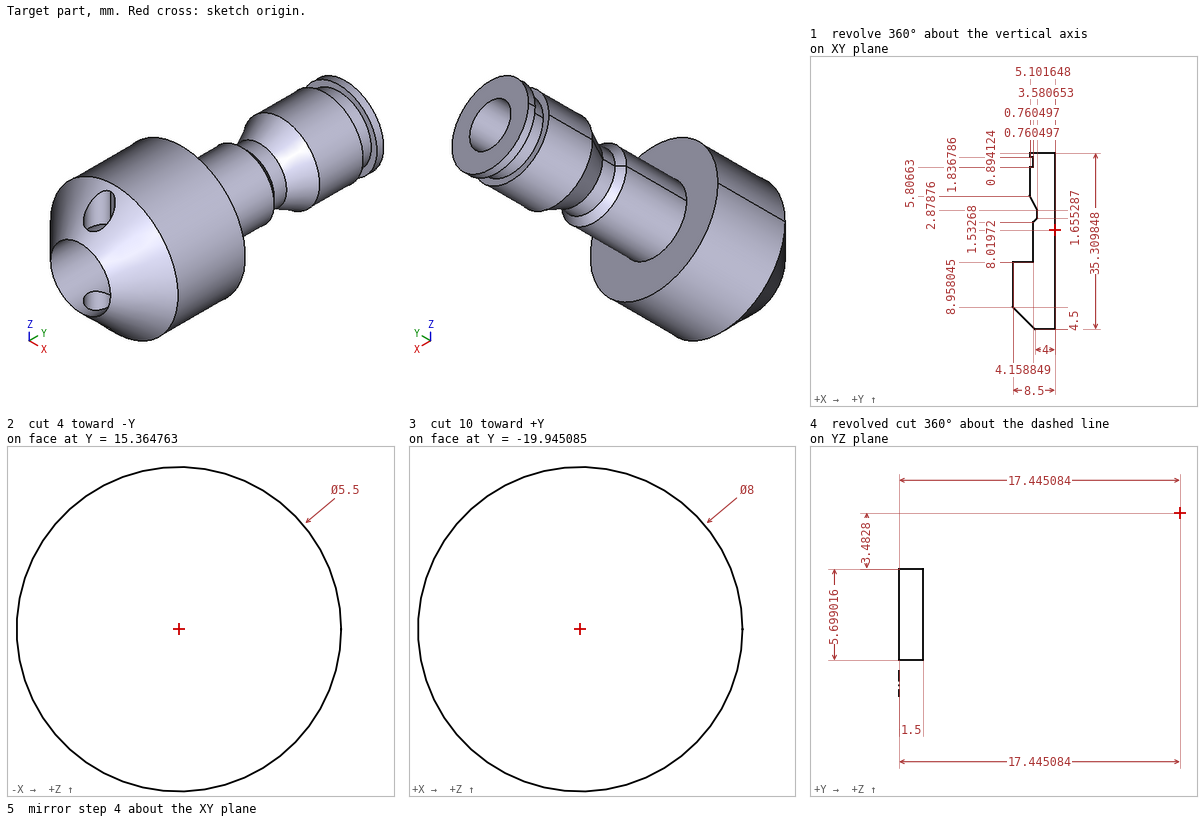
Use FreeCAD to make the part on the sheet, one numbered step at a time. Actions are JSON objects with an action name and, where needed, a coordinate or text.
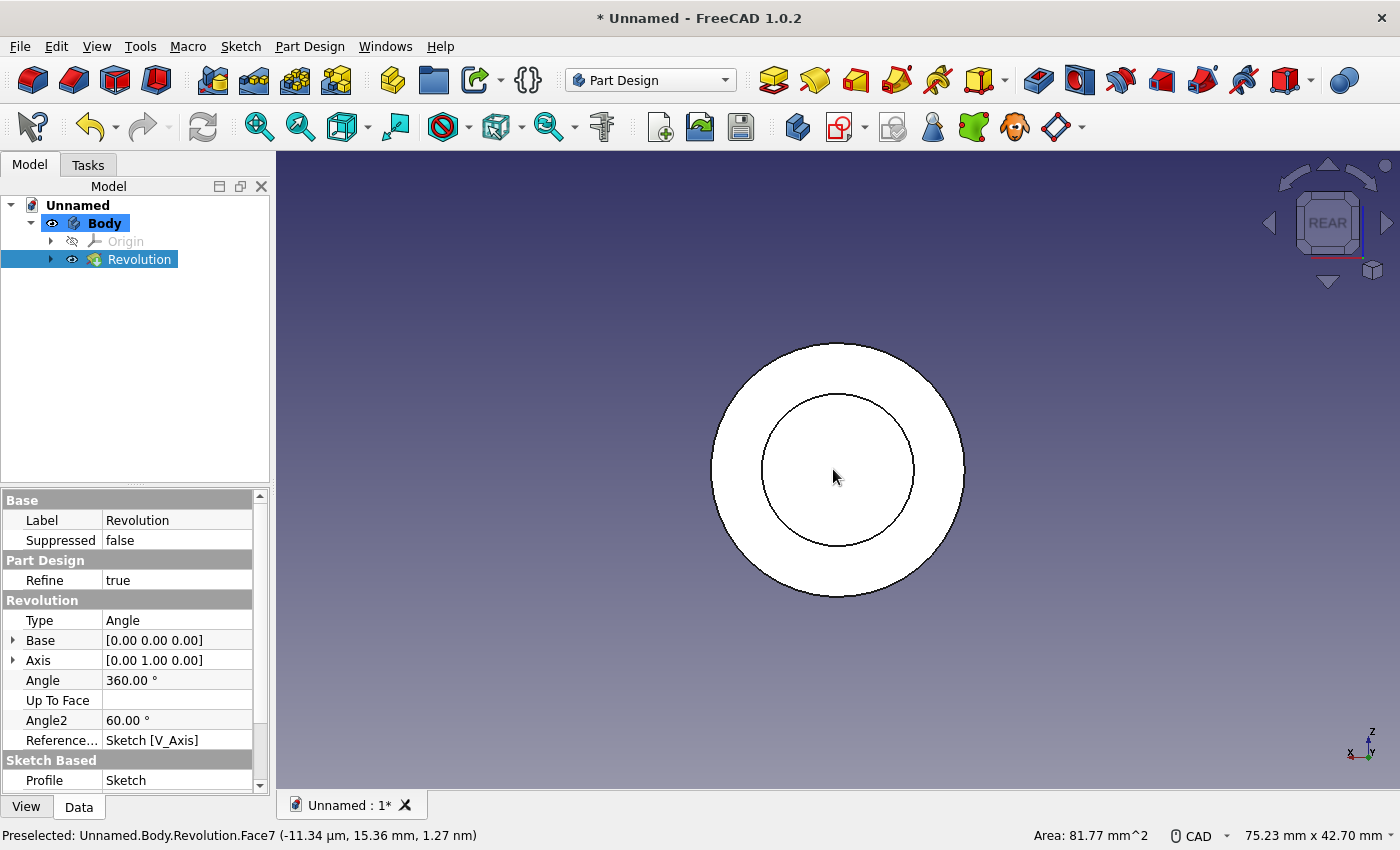
{"action": "left_click", "coordinate": [838, 128]}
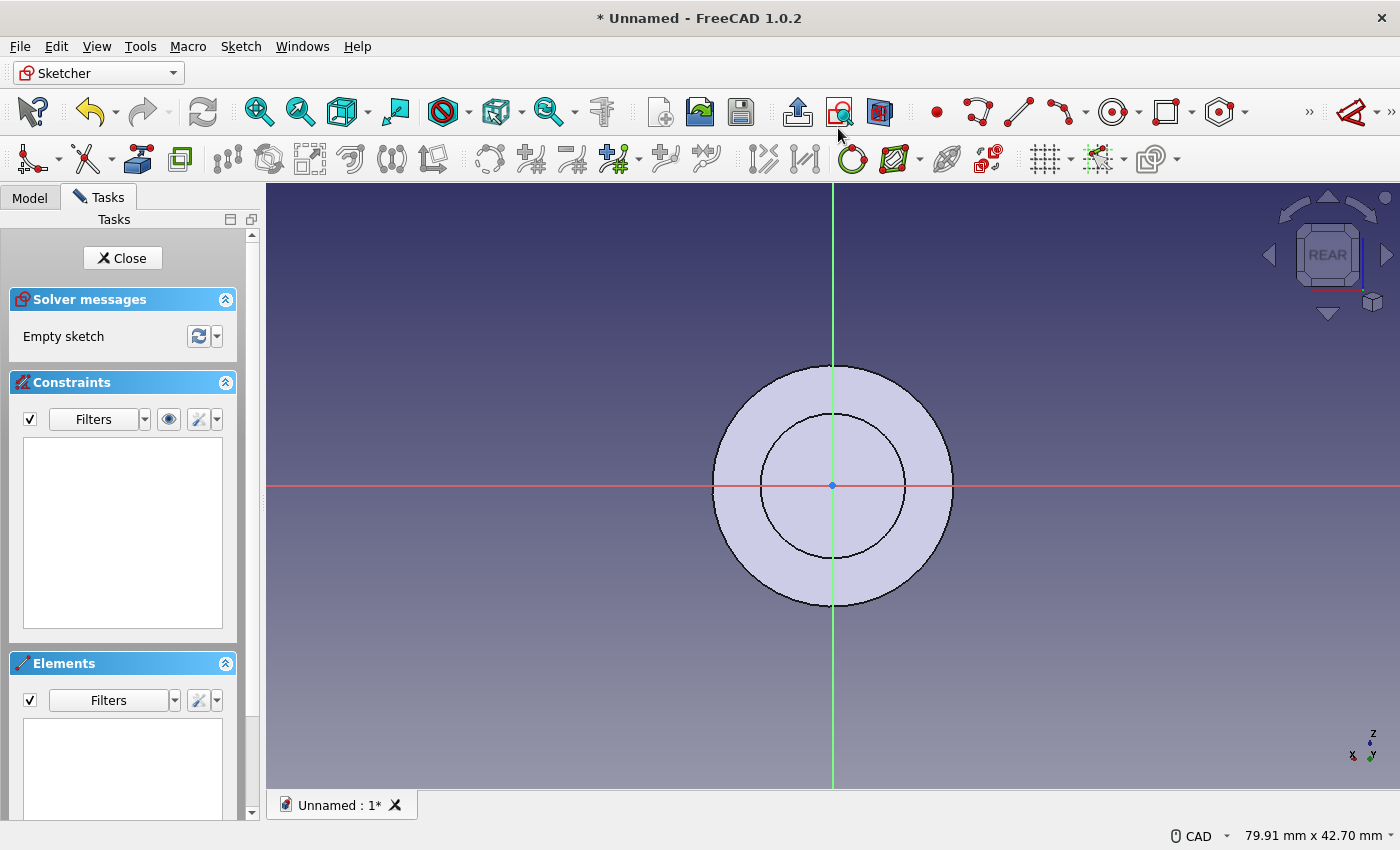
{"action": "scroll", "coordinate": [850, 486], "scroll_direction": "up", "scroll_amount": 8}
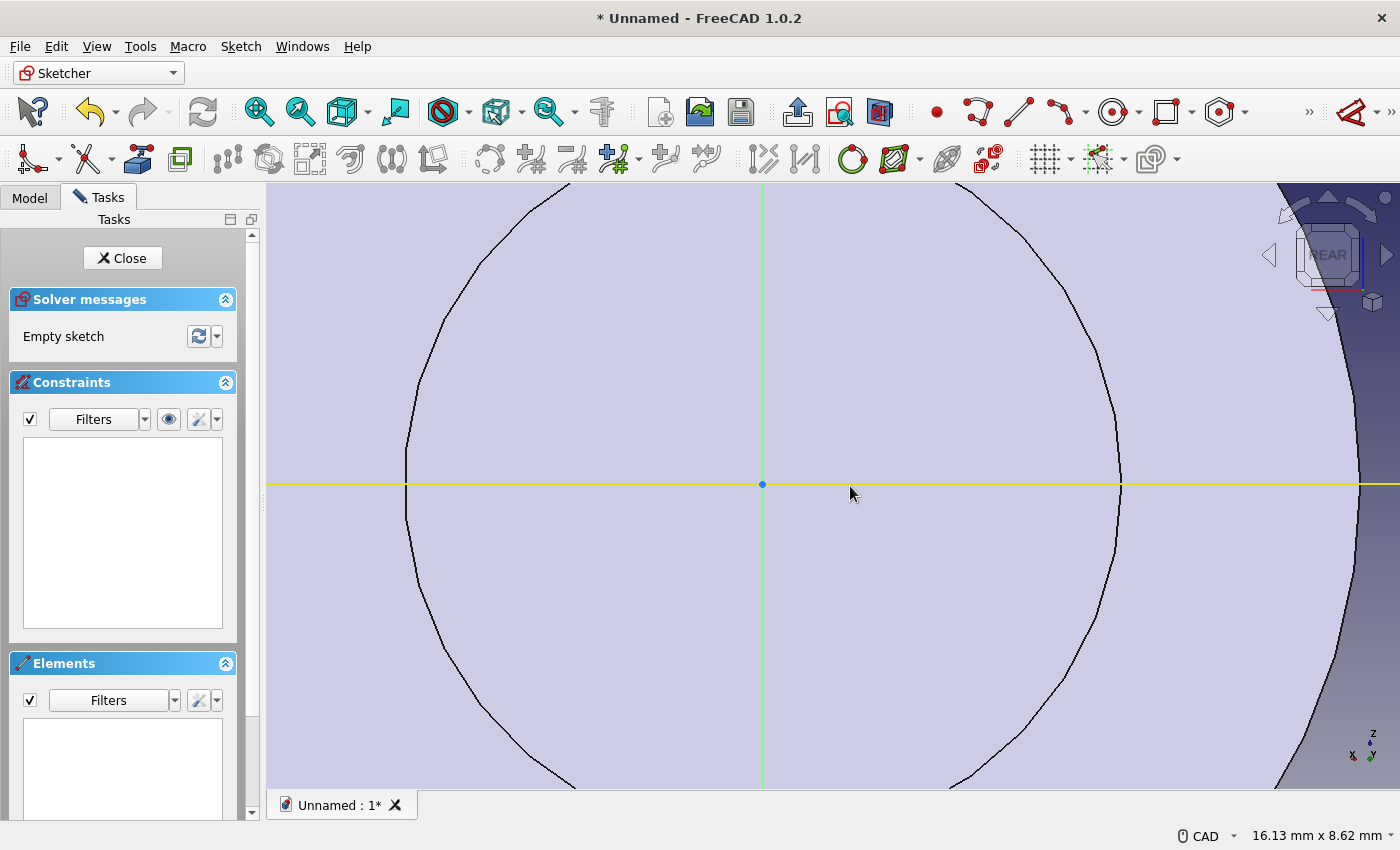
{"action": "left_click", "coordinate": [1112, 112]}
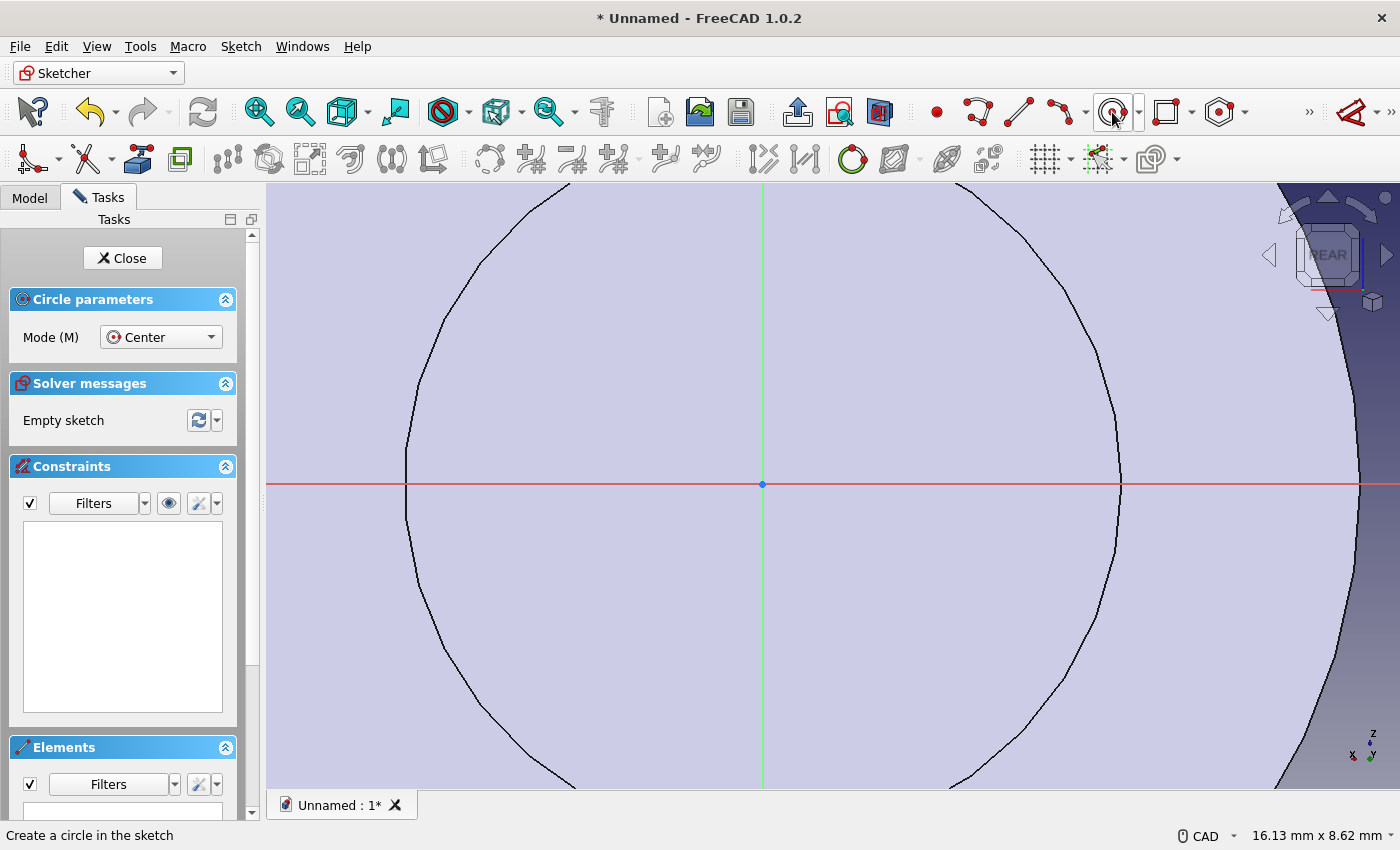
{"action": "left_click", "coordinate": [763, 484]}
{"action": "left_click", "coordinate": [900, 347]}
{"action": "key", "text": "Escape"}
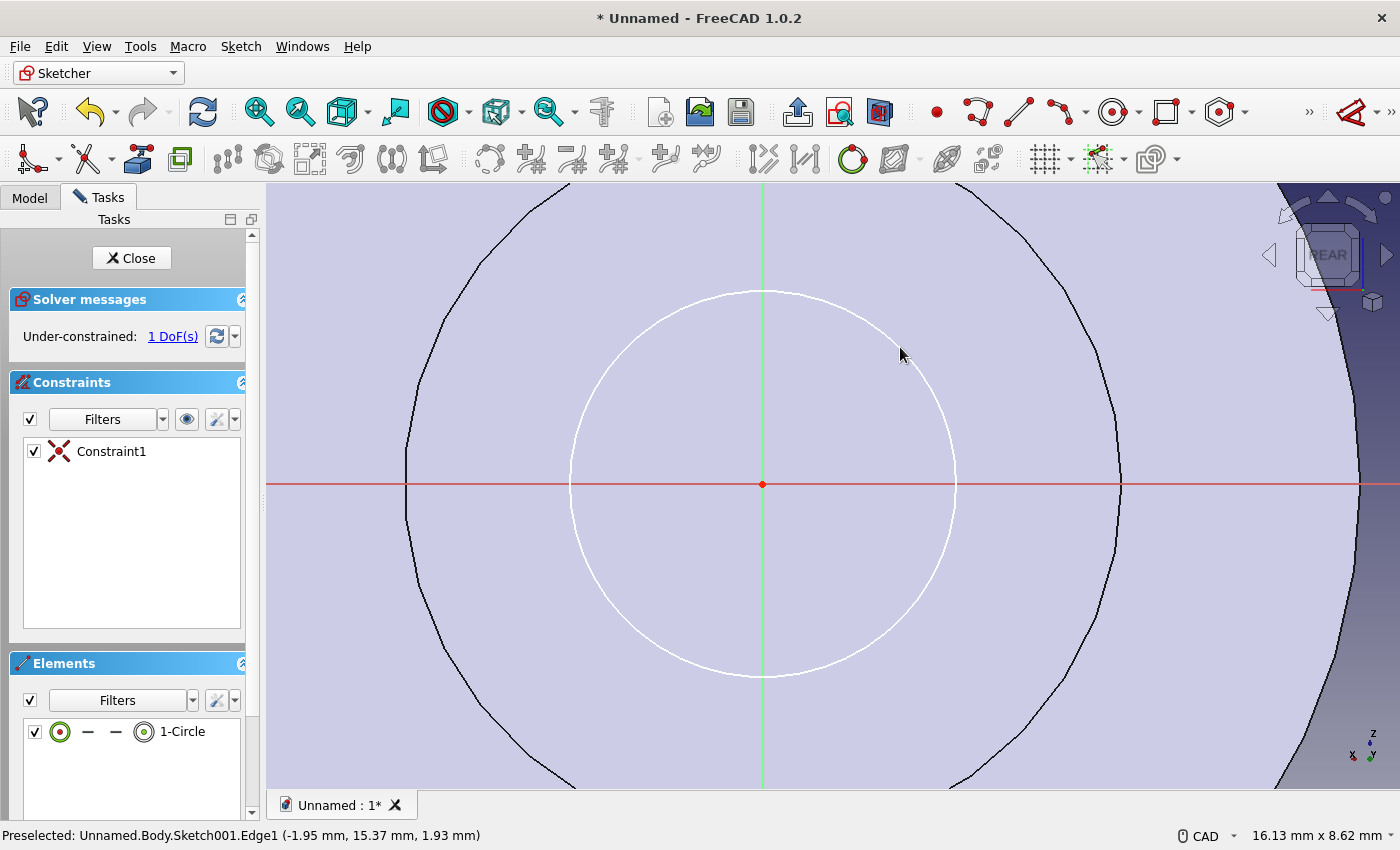
{"action": "key", "text": "d"}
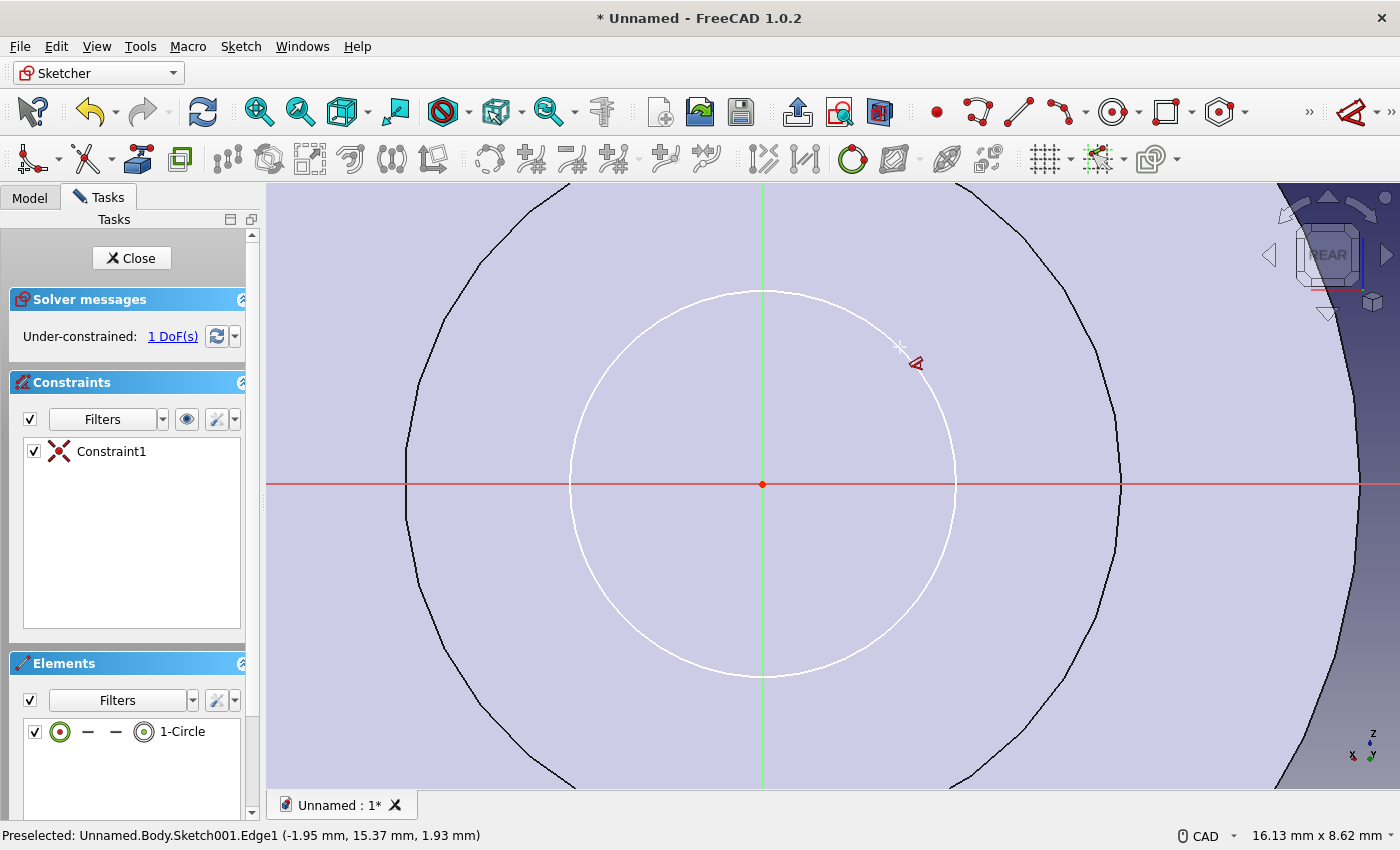
{"action": "left_click", "coordinate": [899, 347]}
{"action": "left_click", "coordinate": [922, 324]}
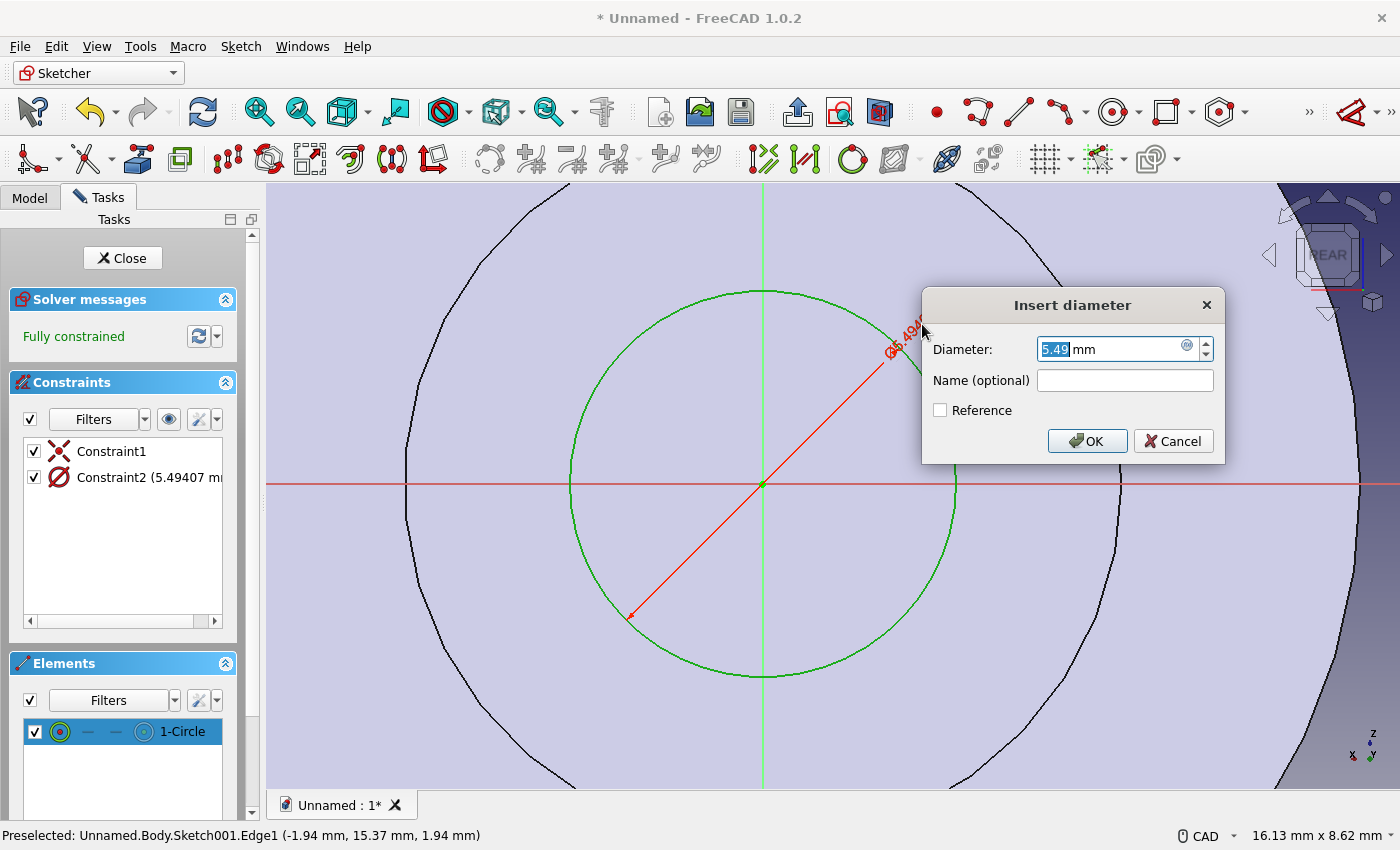
{"action": "type", "text": "5.5"}
{"action": "key", "text": "Return"}
{"action": "key", "text": "Escape"}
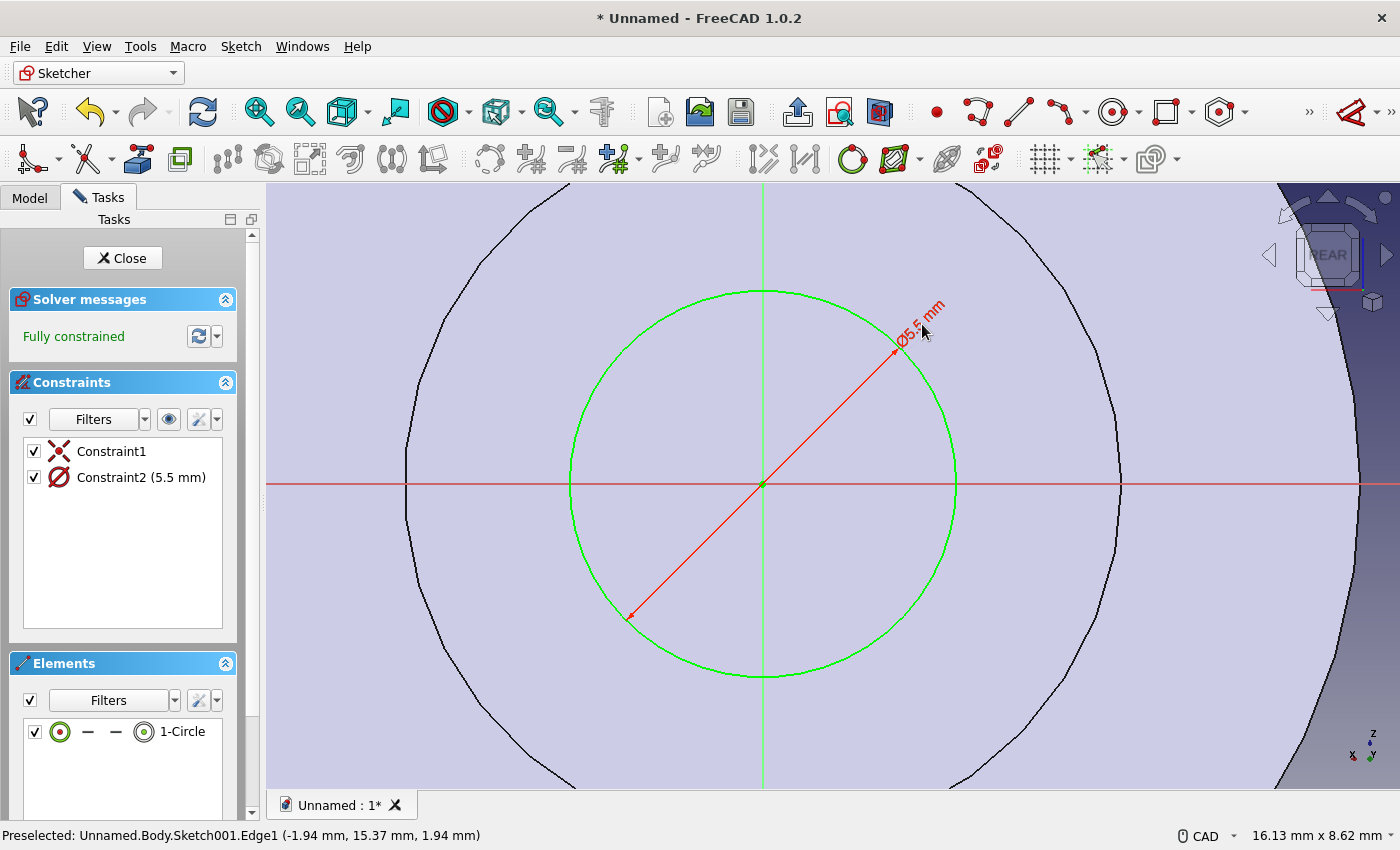
{"action": "left_click", "coordinate": [123, 258]}